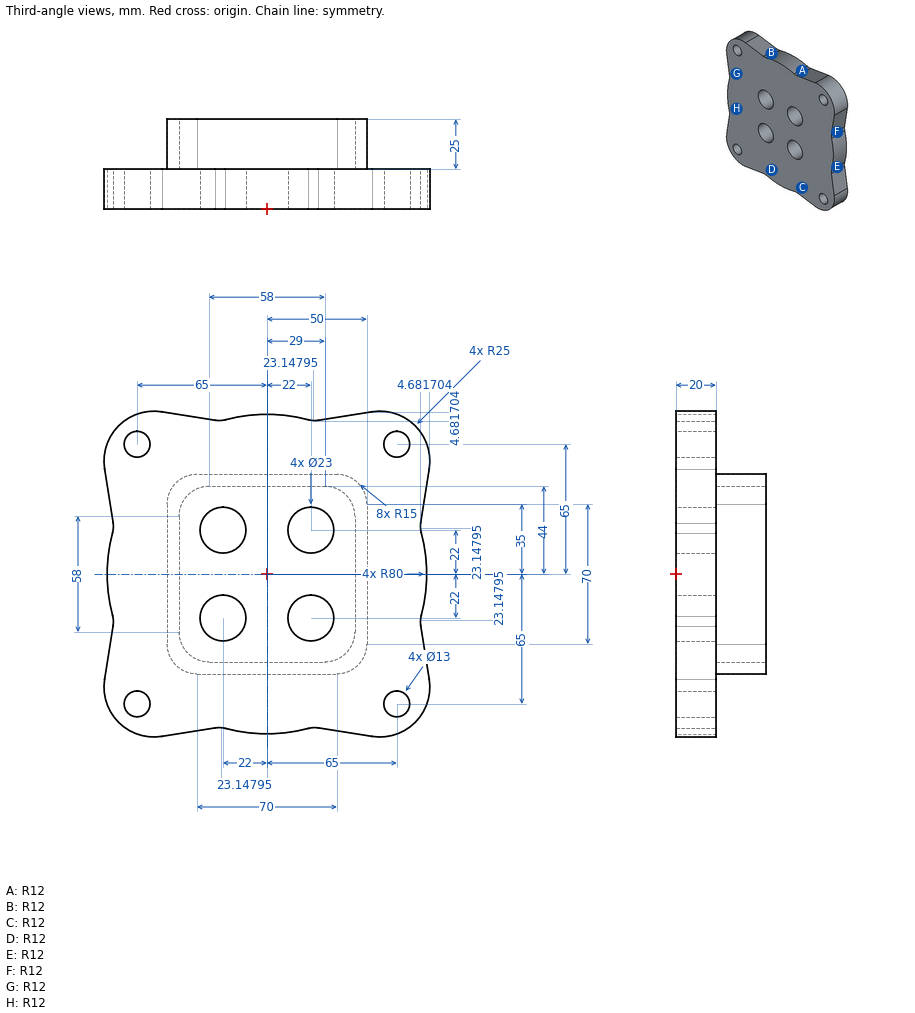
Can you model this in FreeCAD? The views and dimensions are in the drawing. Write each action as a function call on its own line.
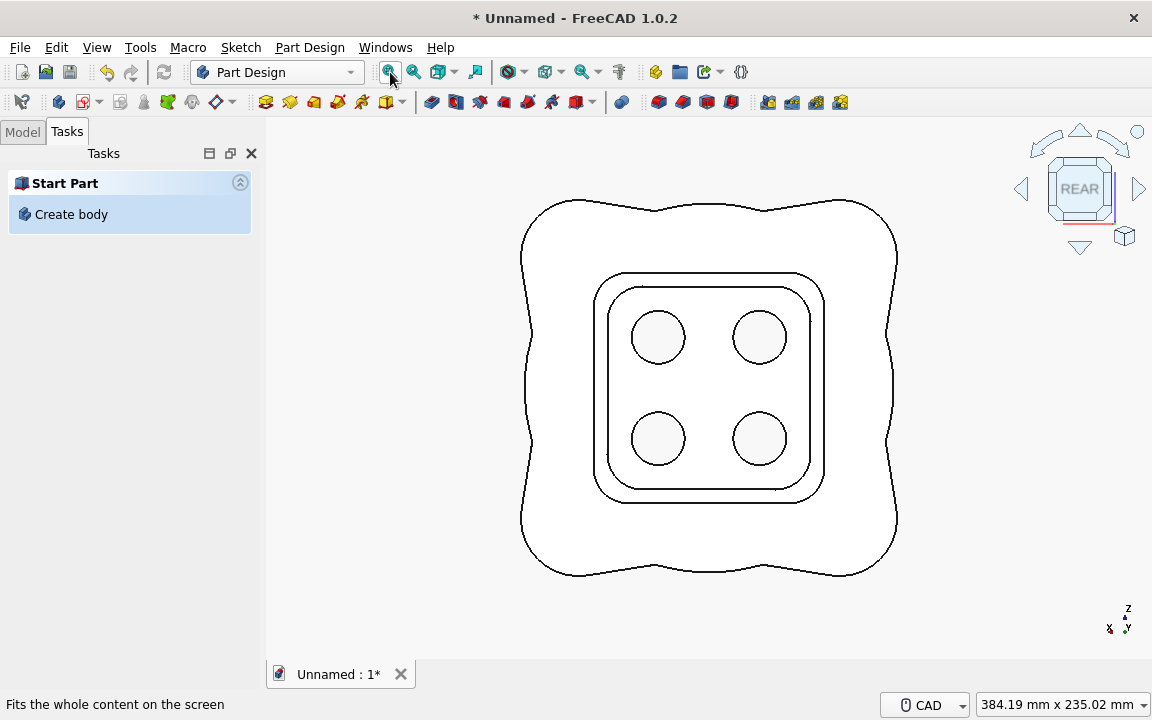
key(6)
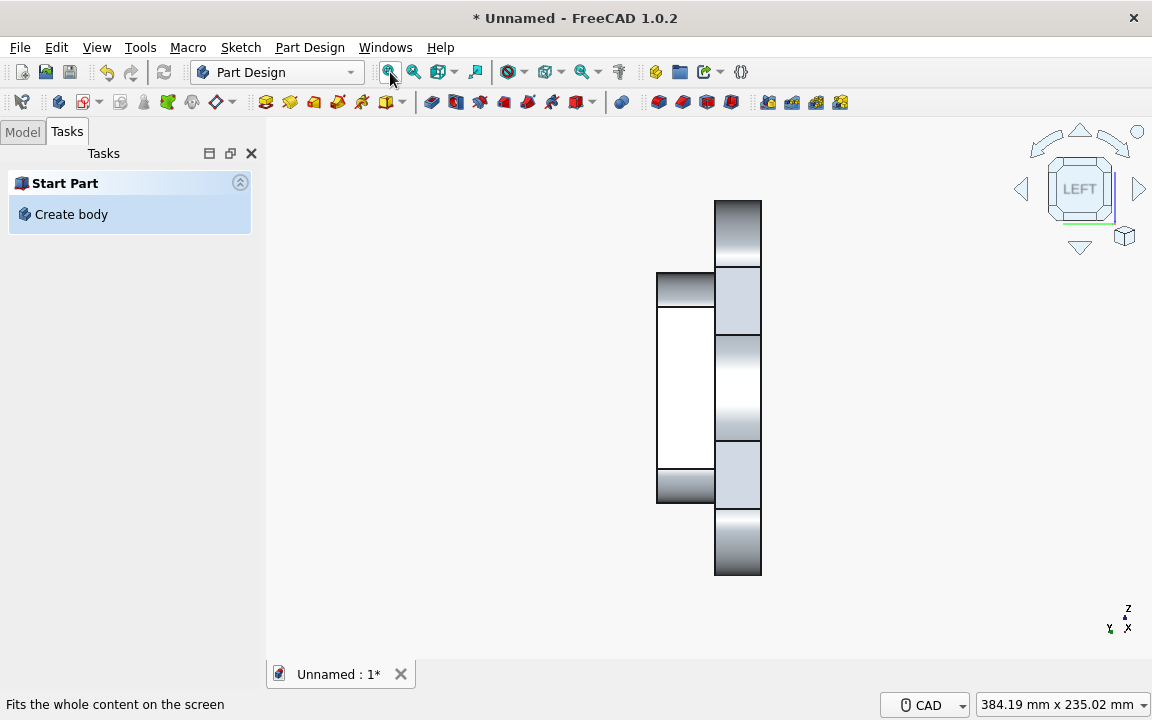
key(v)
key(3)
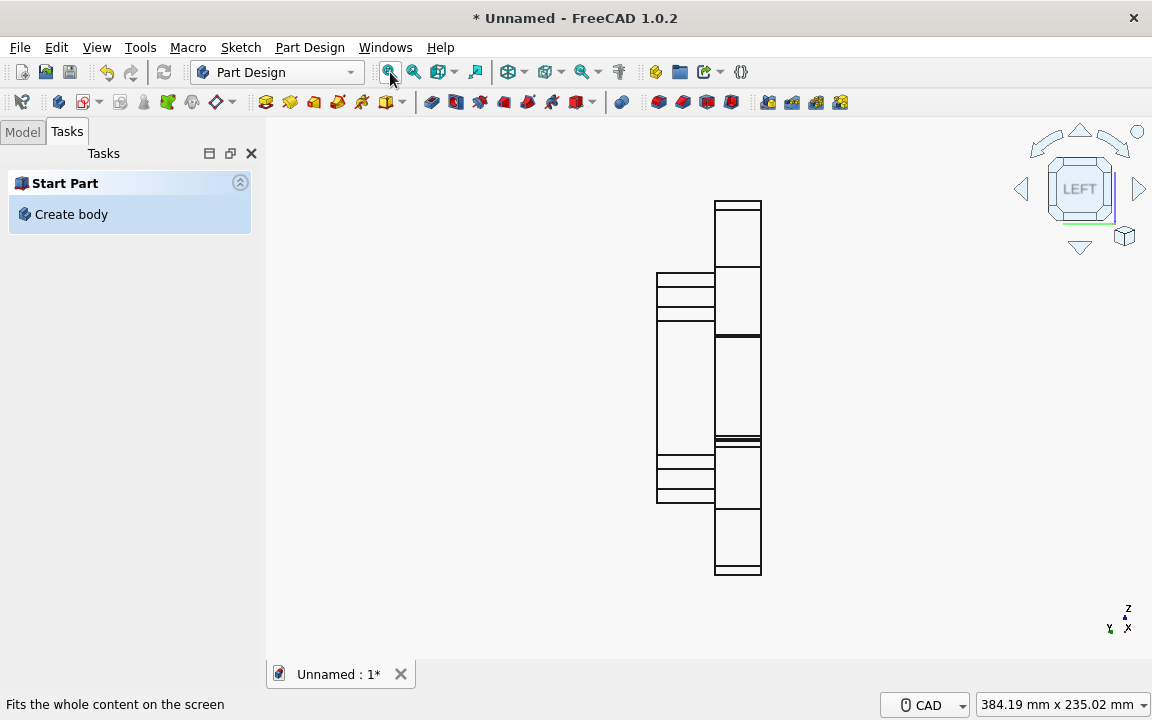
key(0)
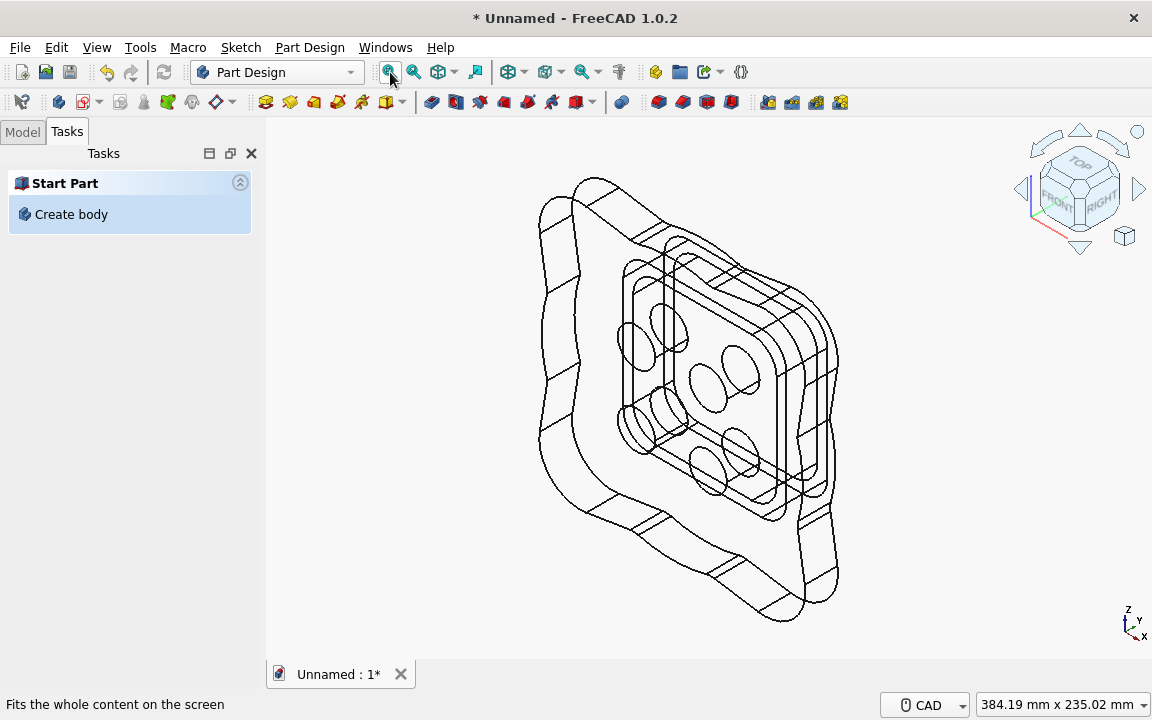
click(813, 427)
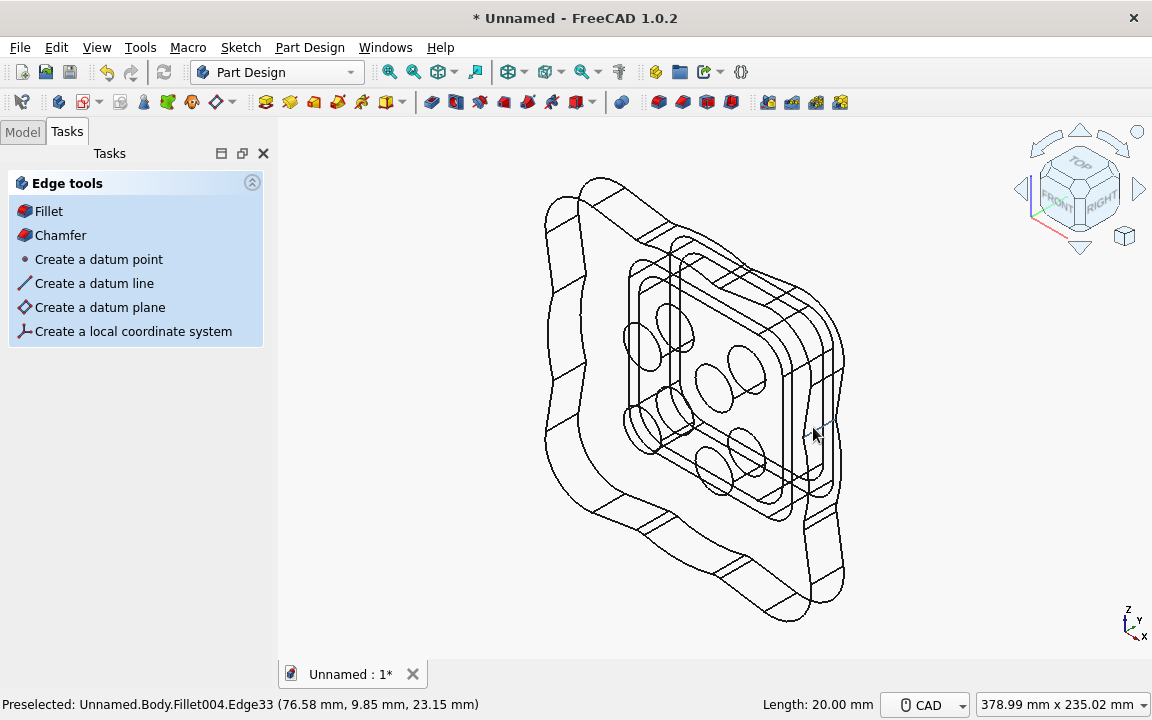
key(v)
key(1)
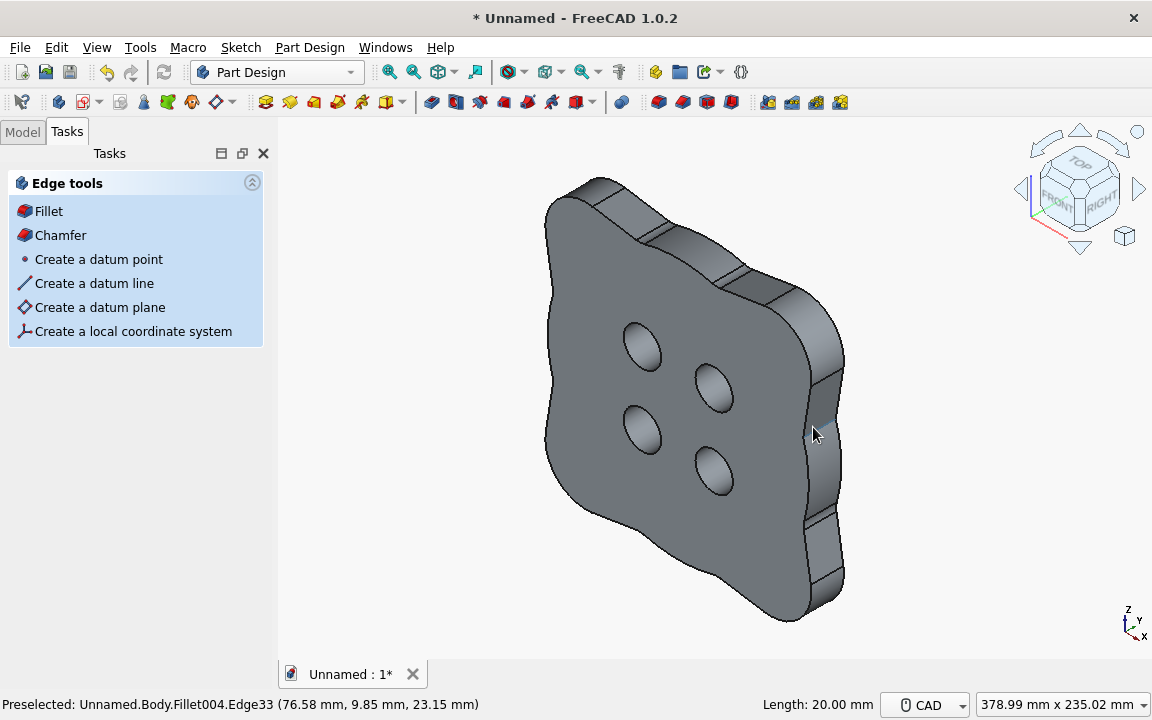
click(660, 102)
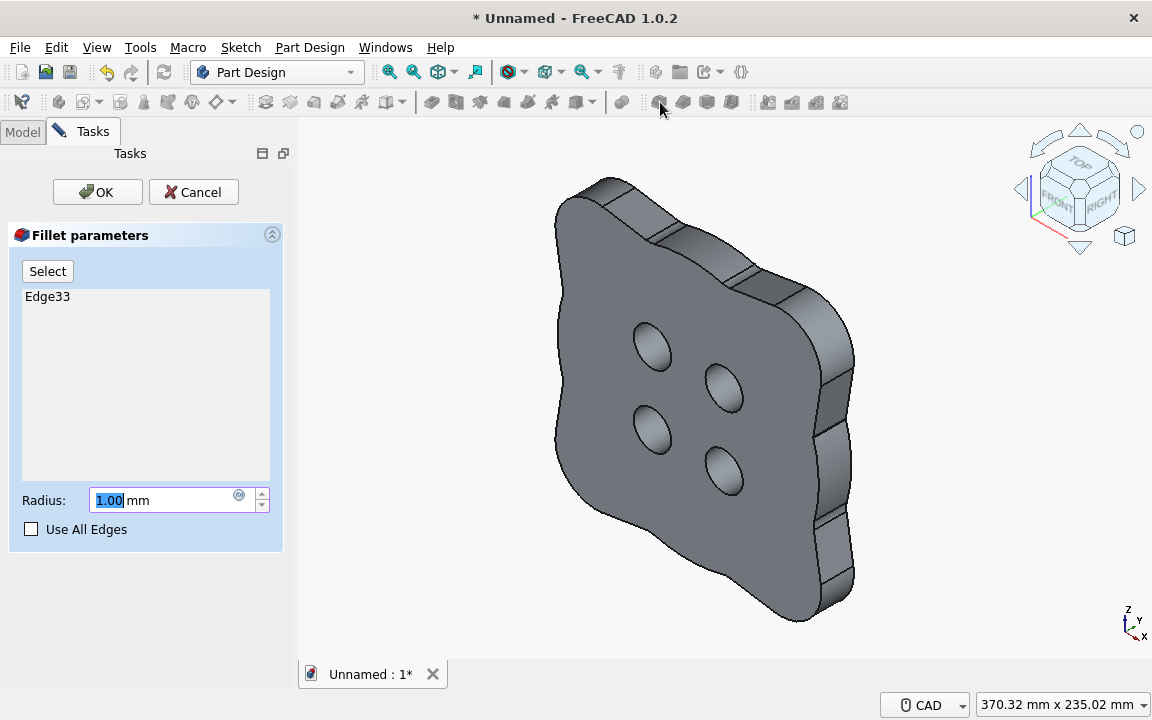
text(12)
key(Tab)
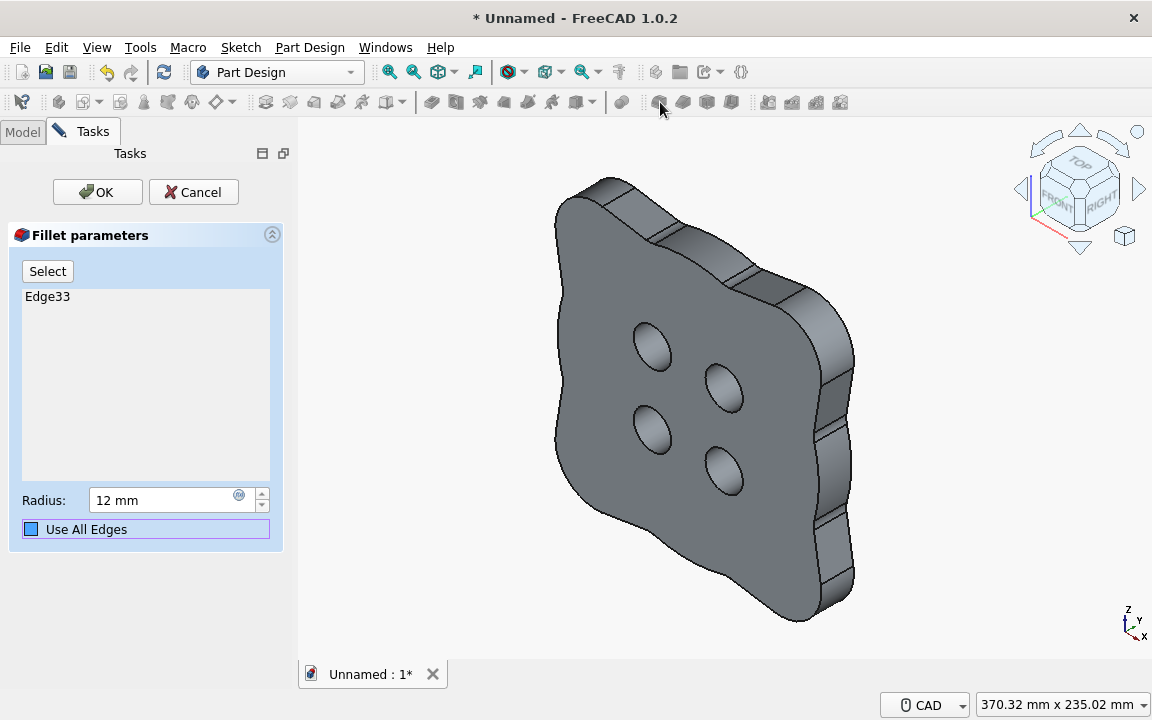
click(98, 192)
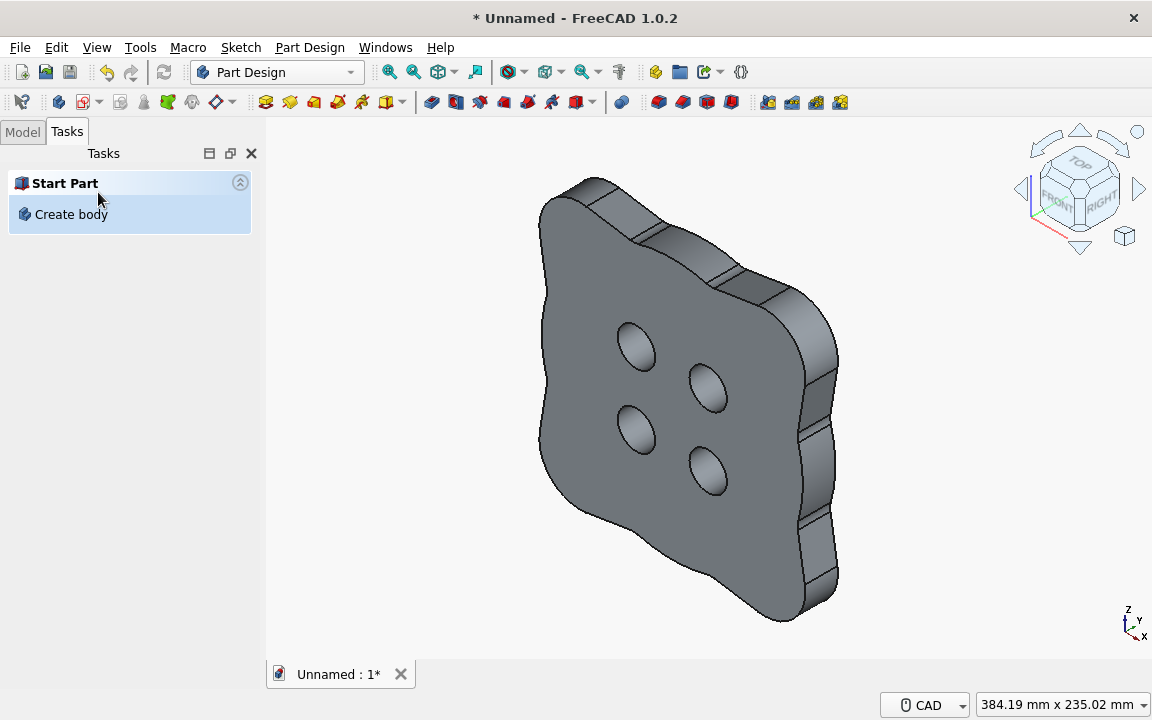
key(2)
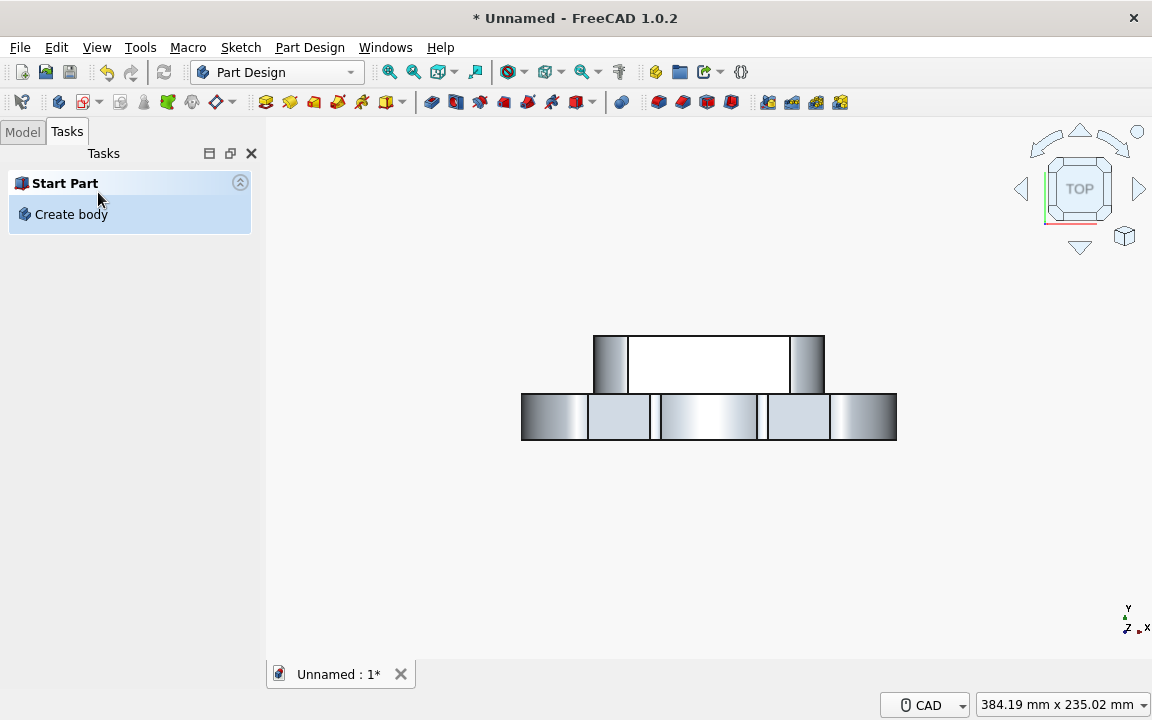
click(390, 72)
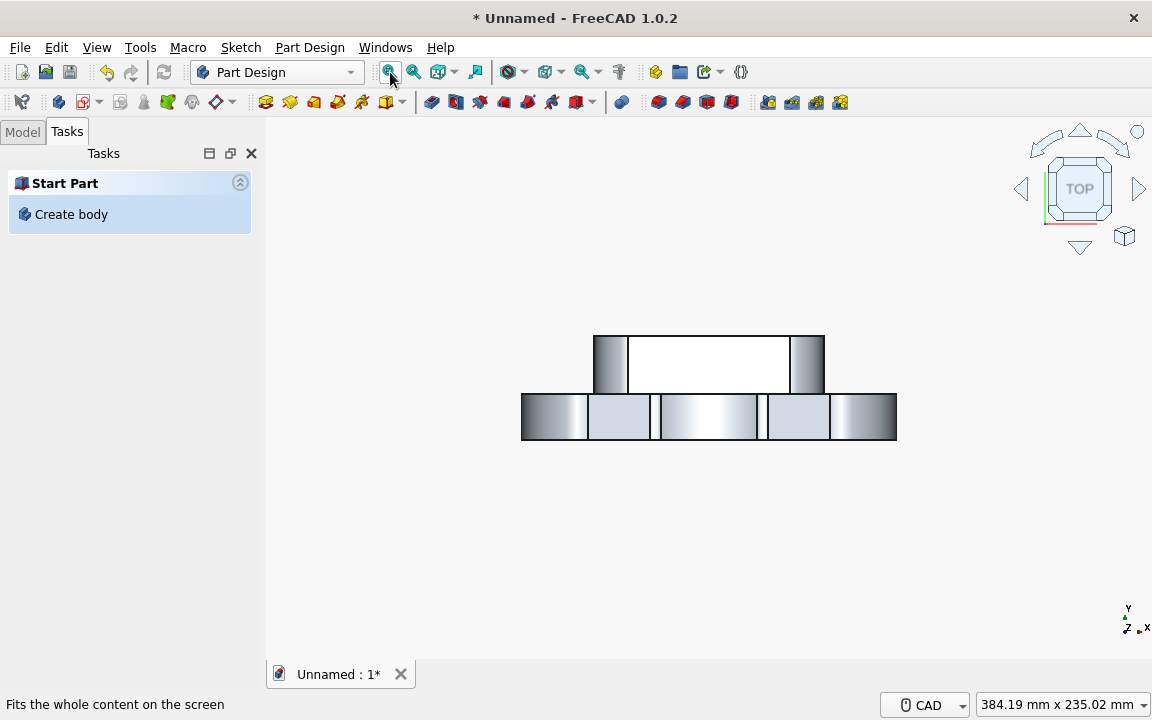
key(0)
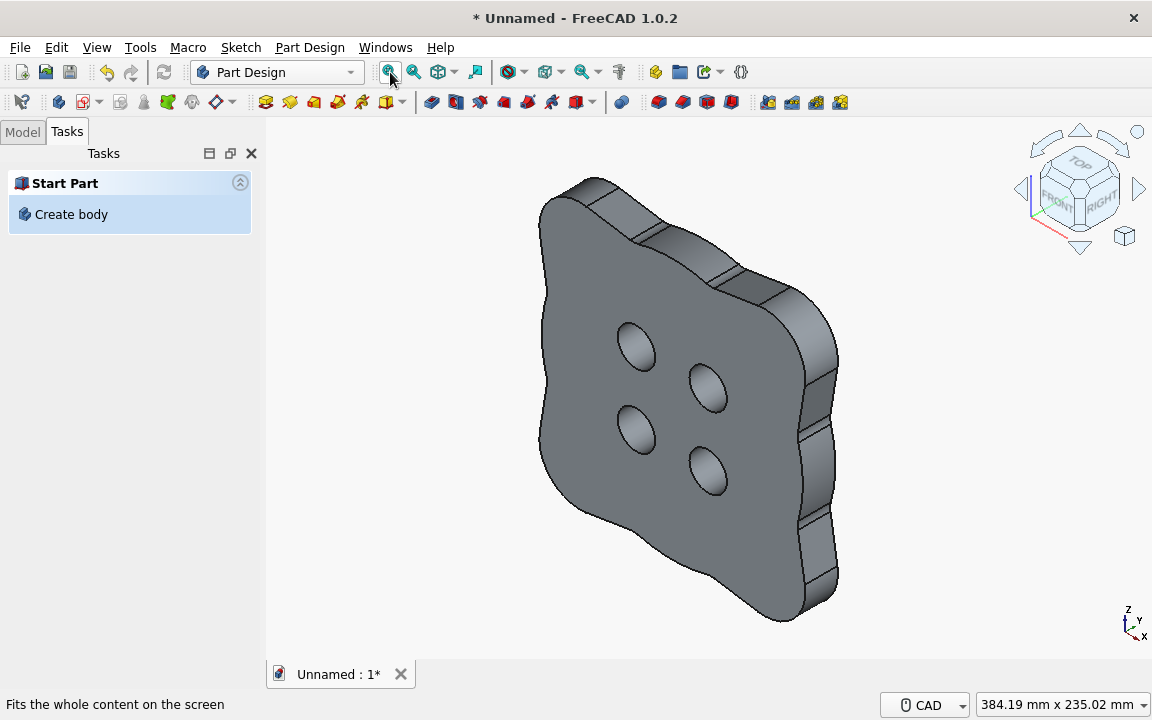
key(1)